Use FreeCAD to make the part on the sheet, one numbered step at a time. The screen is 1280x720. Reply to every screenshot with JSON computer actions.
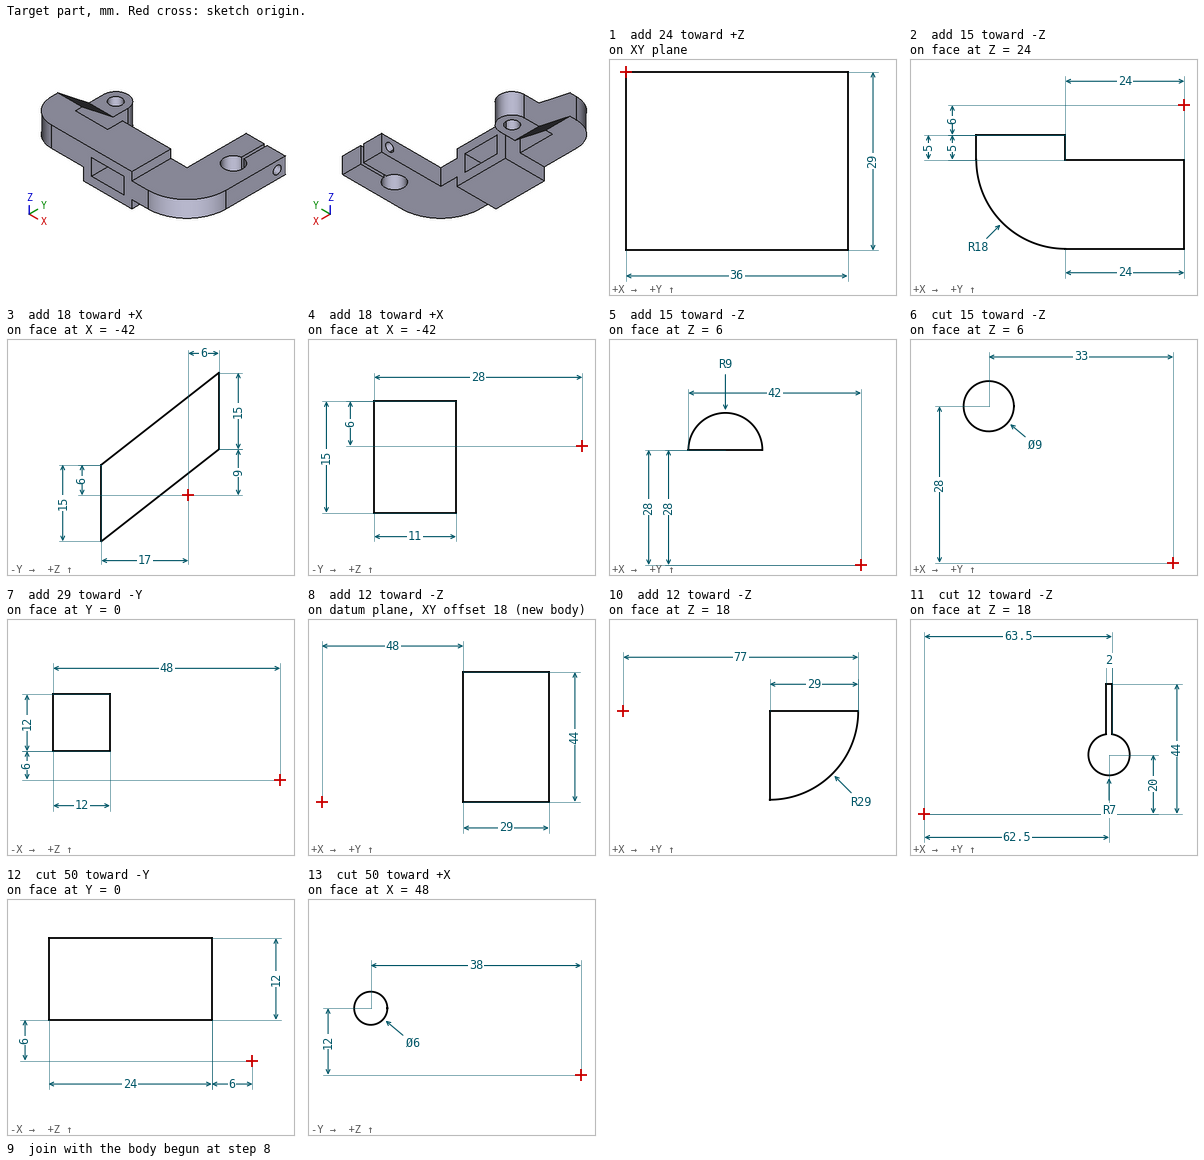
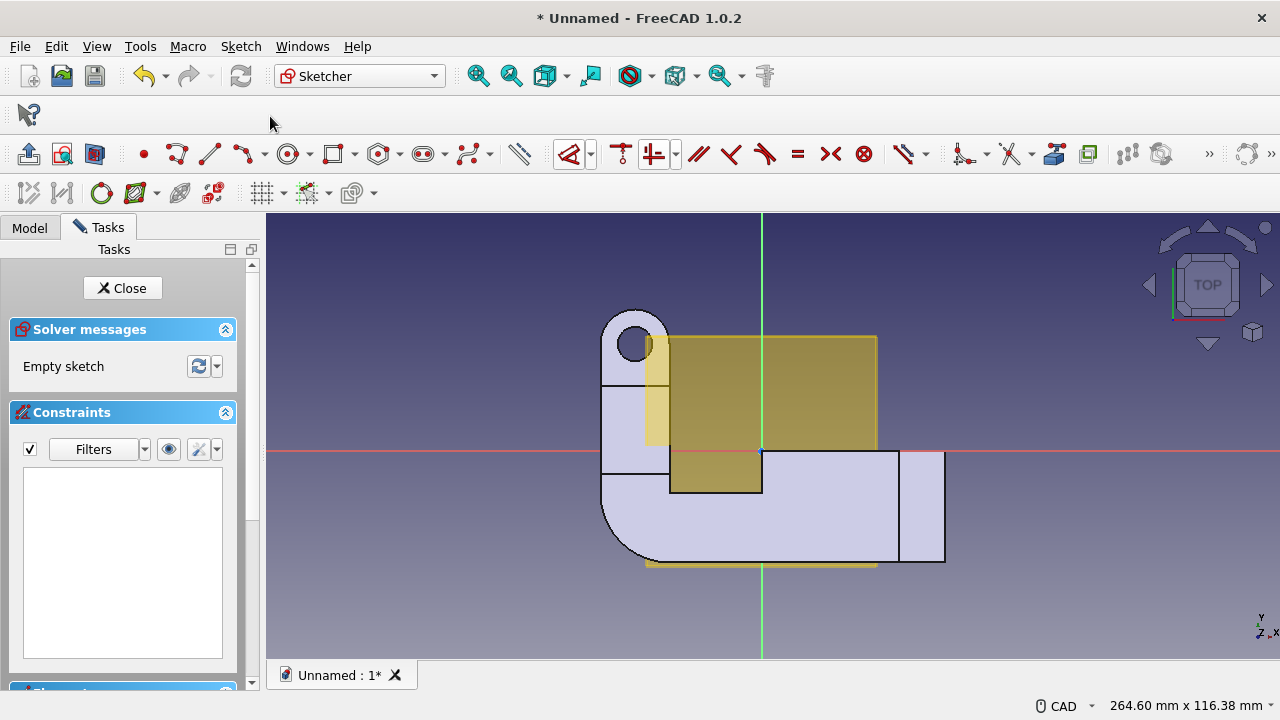
{"action": "scroll", "coordinate": [1115, 241], "scroll_direction": "up", "scroll_amount": 2}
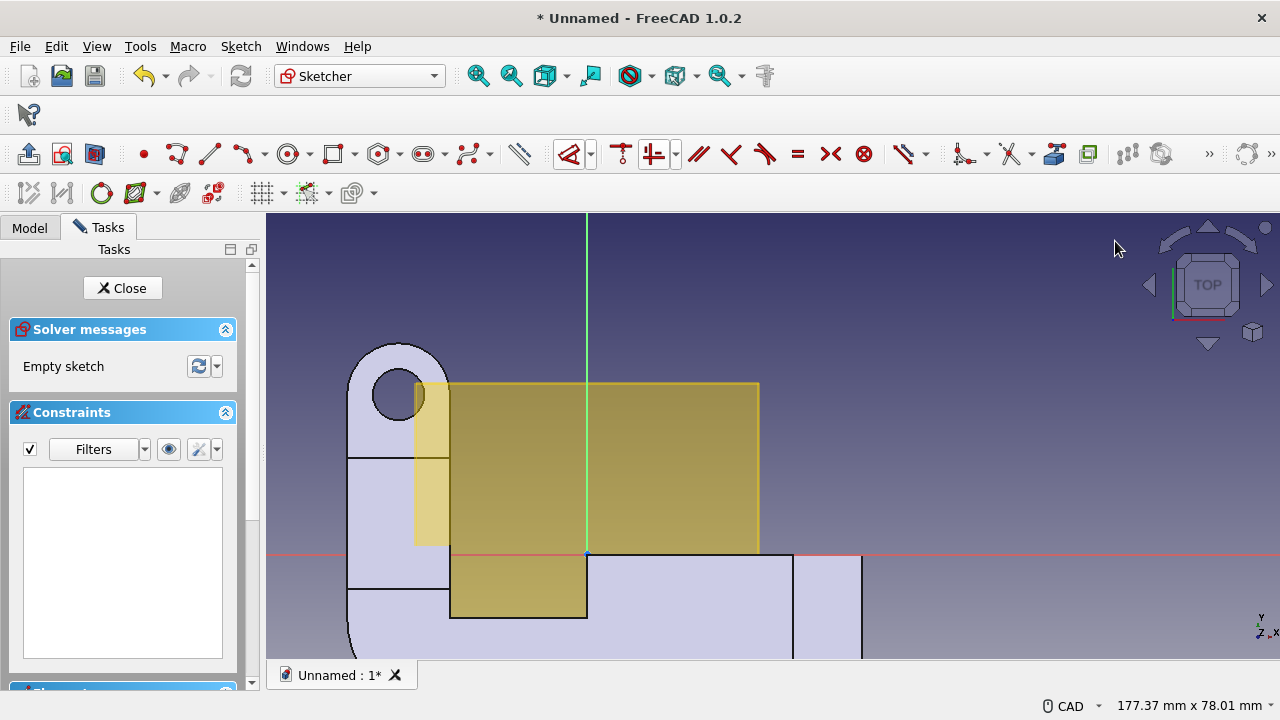
{"action": "left_click", "coordinate": [332, 154]}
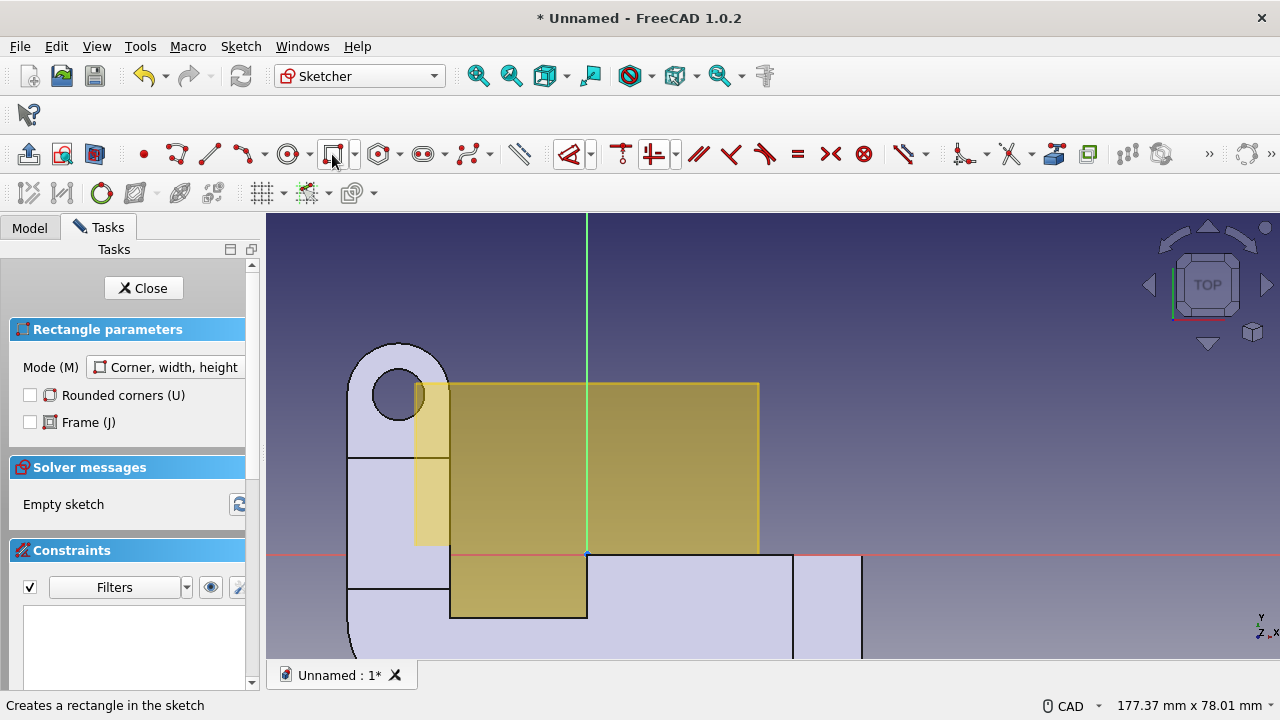
{"action": "left_click", "coordinate": [862, 303]}
{"action": "left_click", "coordinate": [1027, 555]}
{"action": "key", "text": "Escape"}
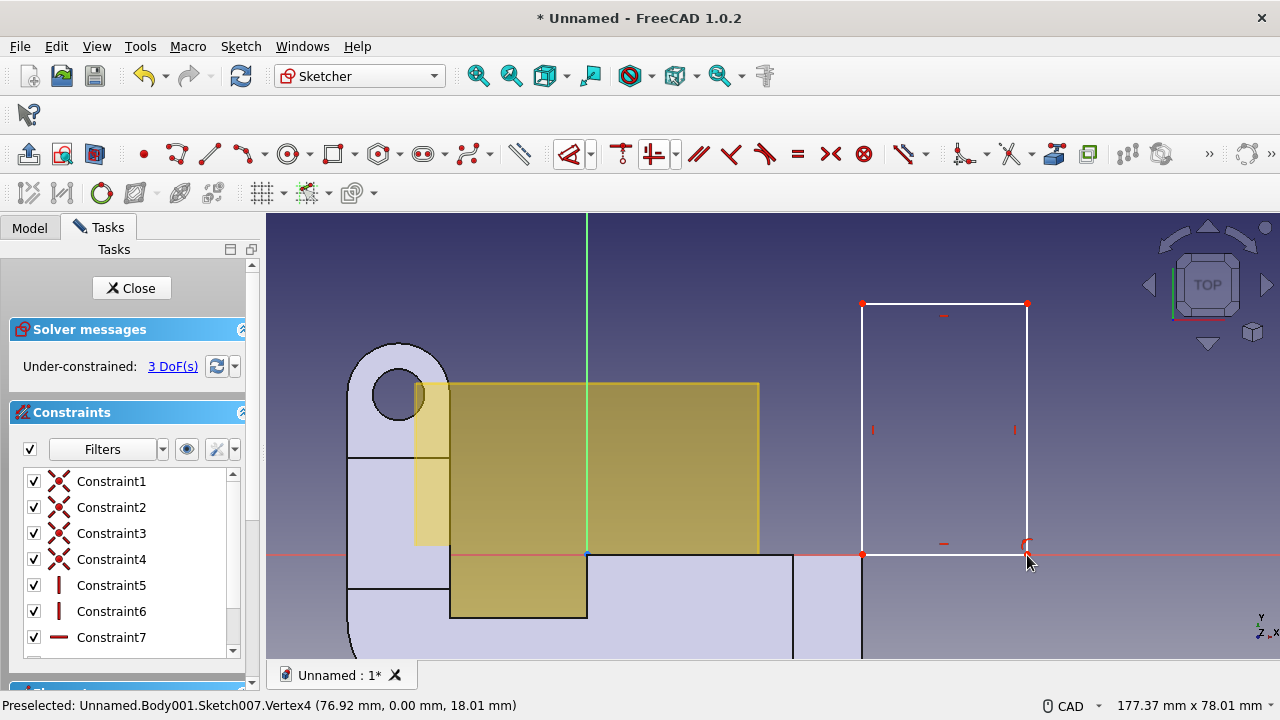
{"action": "left_click", "coordinate": [862, 379]}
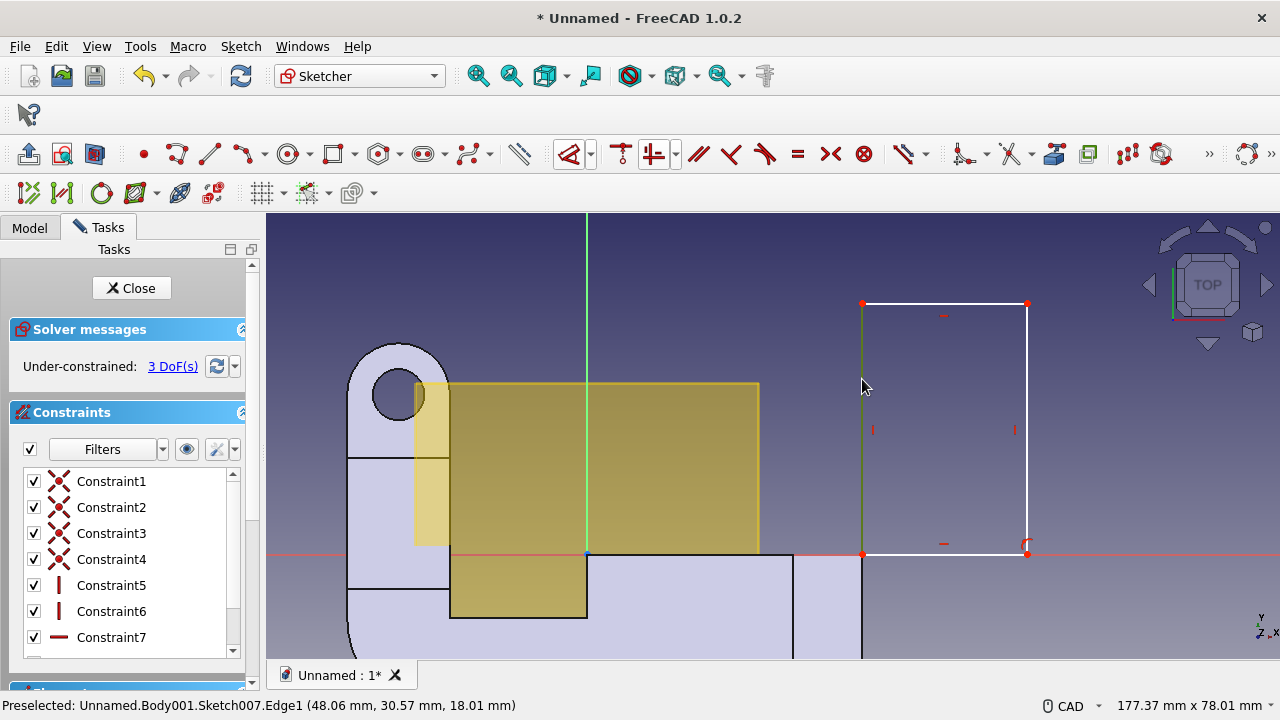
{"action": "key", "text": "i"}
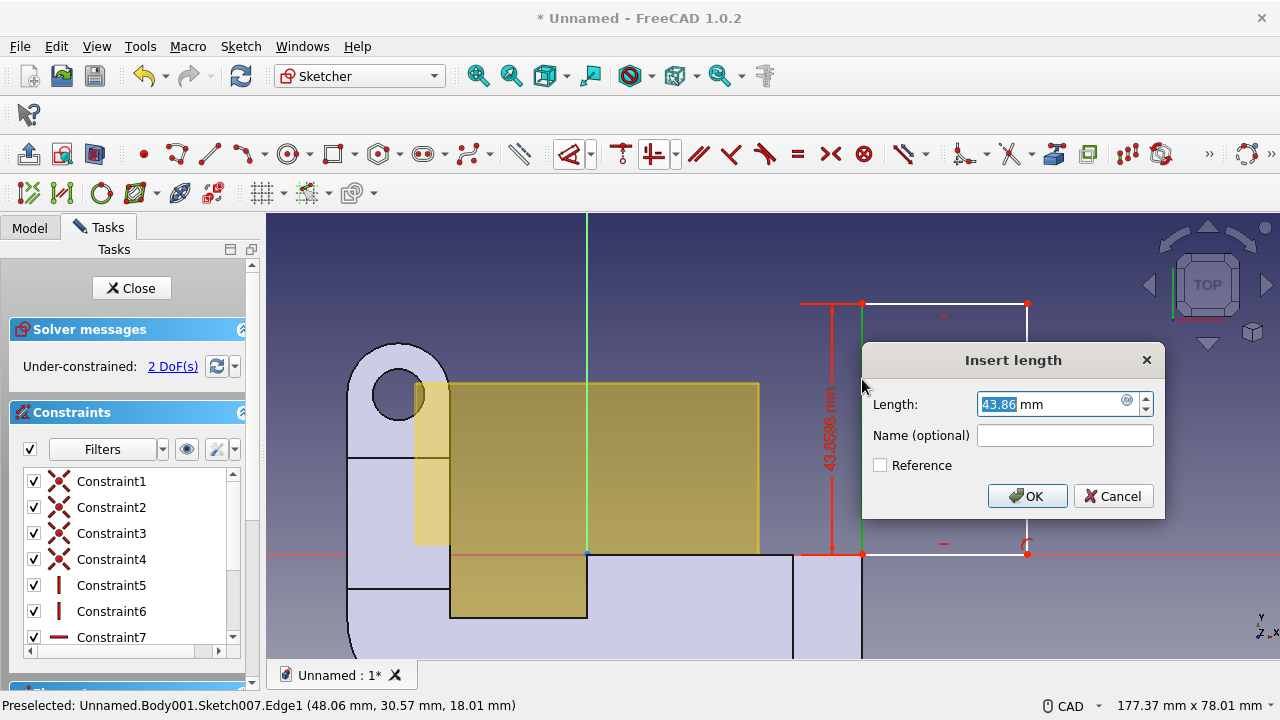
{"action": "type", "text": "44"}
{"action": "key", "text": "Return"}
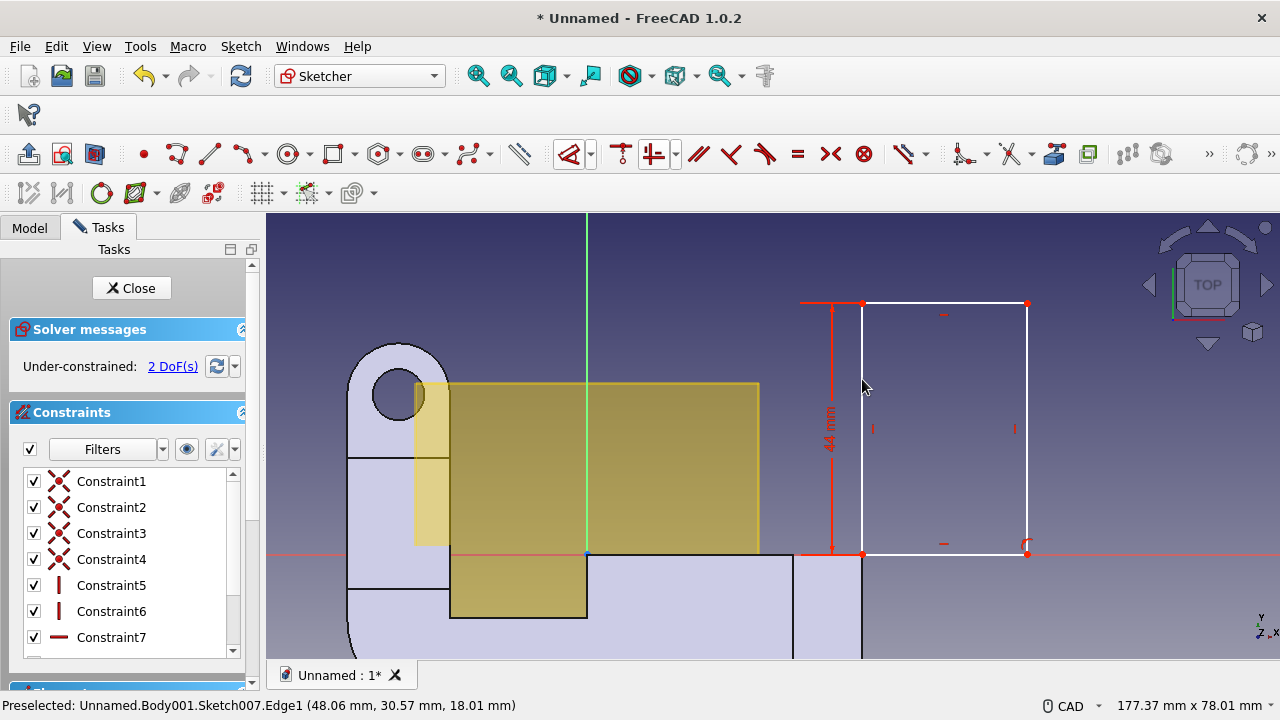
{"action": "left_click", "coordinate": [911, 555]}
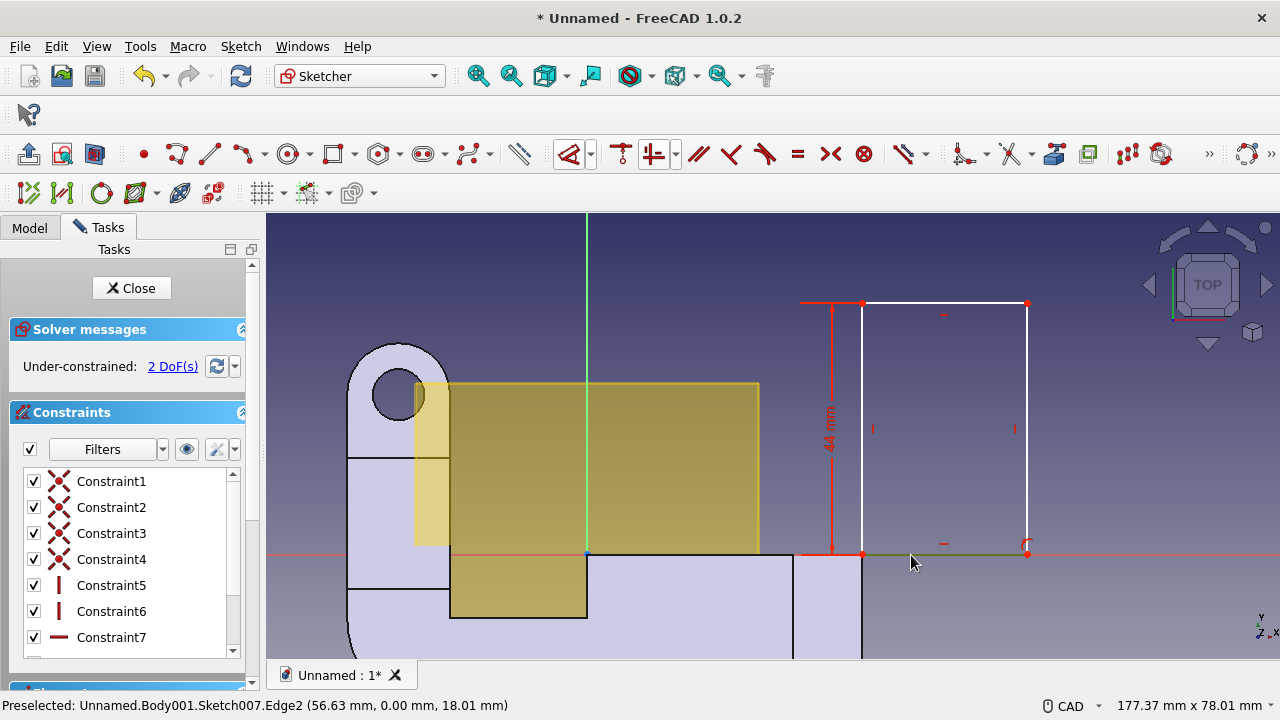
{"action": "left_click", "coordinate": [590, 154]}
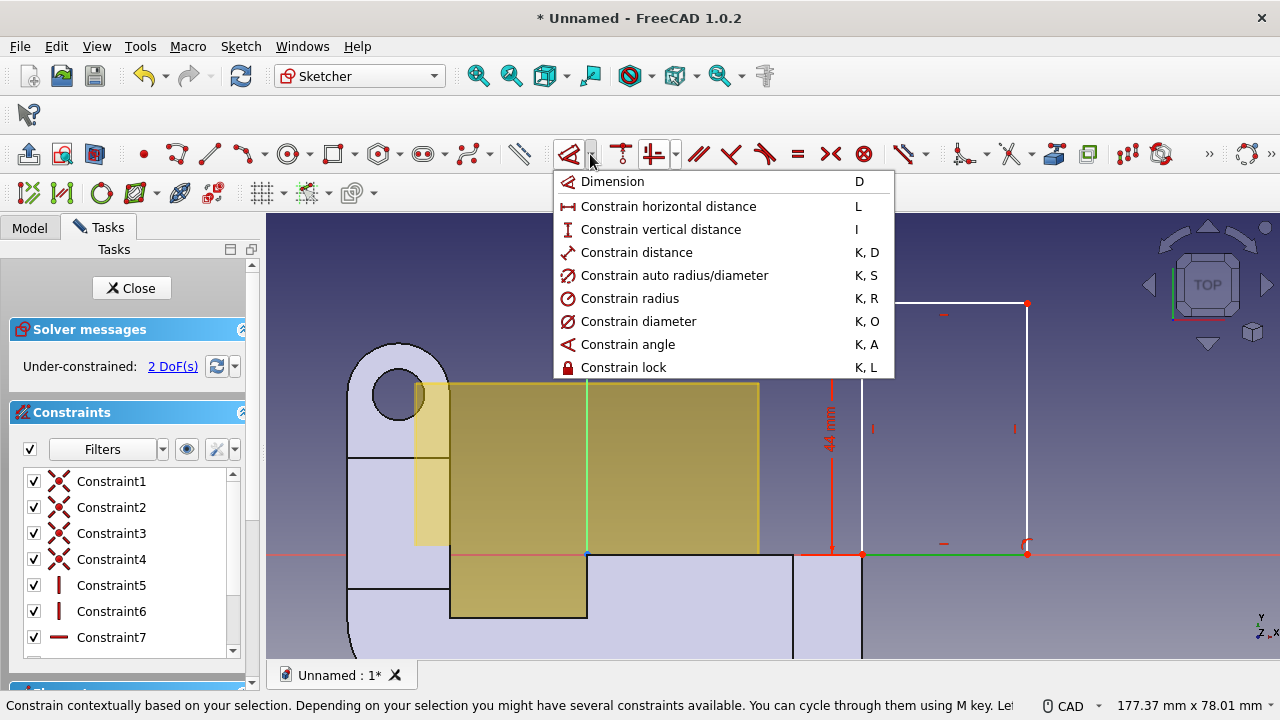
{"action": "left_click", "coordinate": [724, 206]}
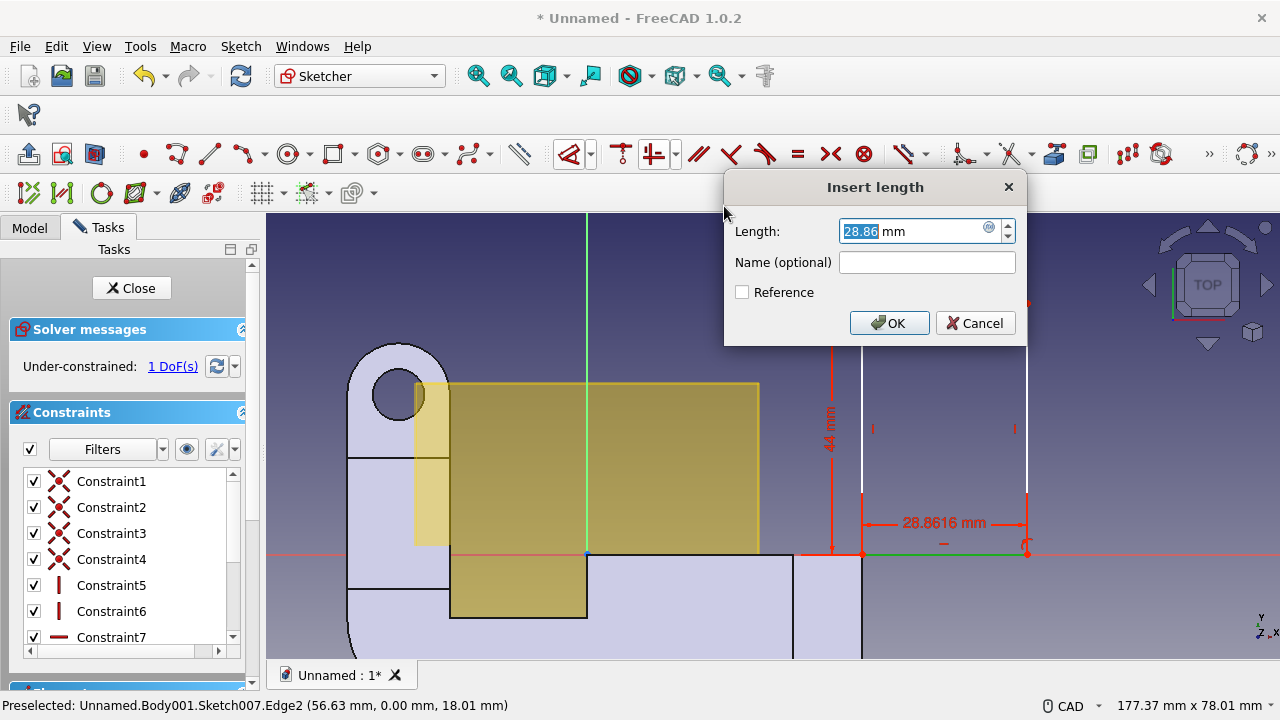
{"action": "type", "text": "29"}
{"action": "key", "text": "Return"}